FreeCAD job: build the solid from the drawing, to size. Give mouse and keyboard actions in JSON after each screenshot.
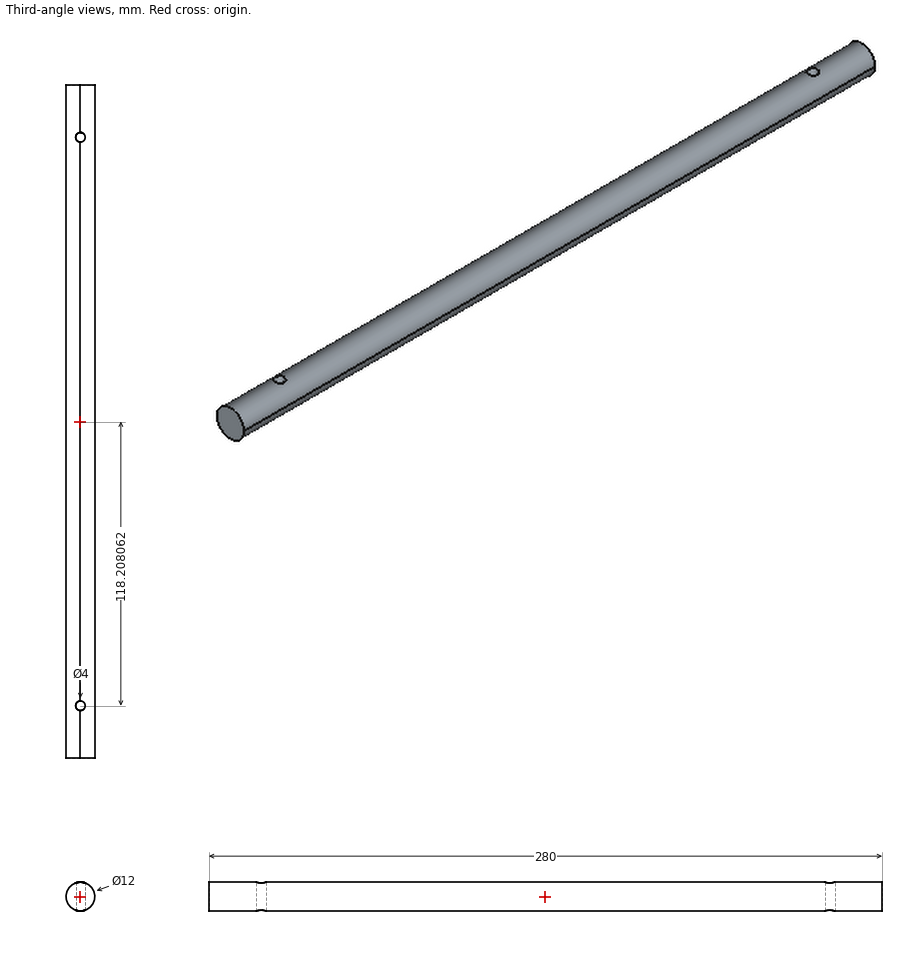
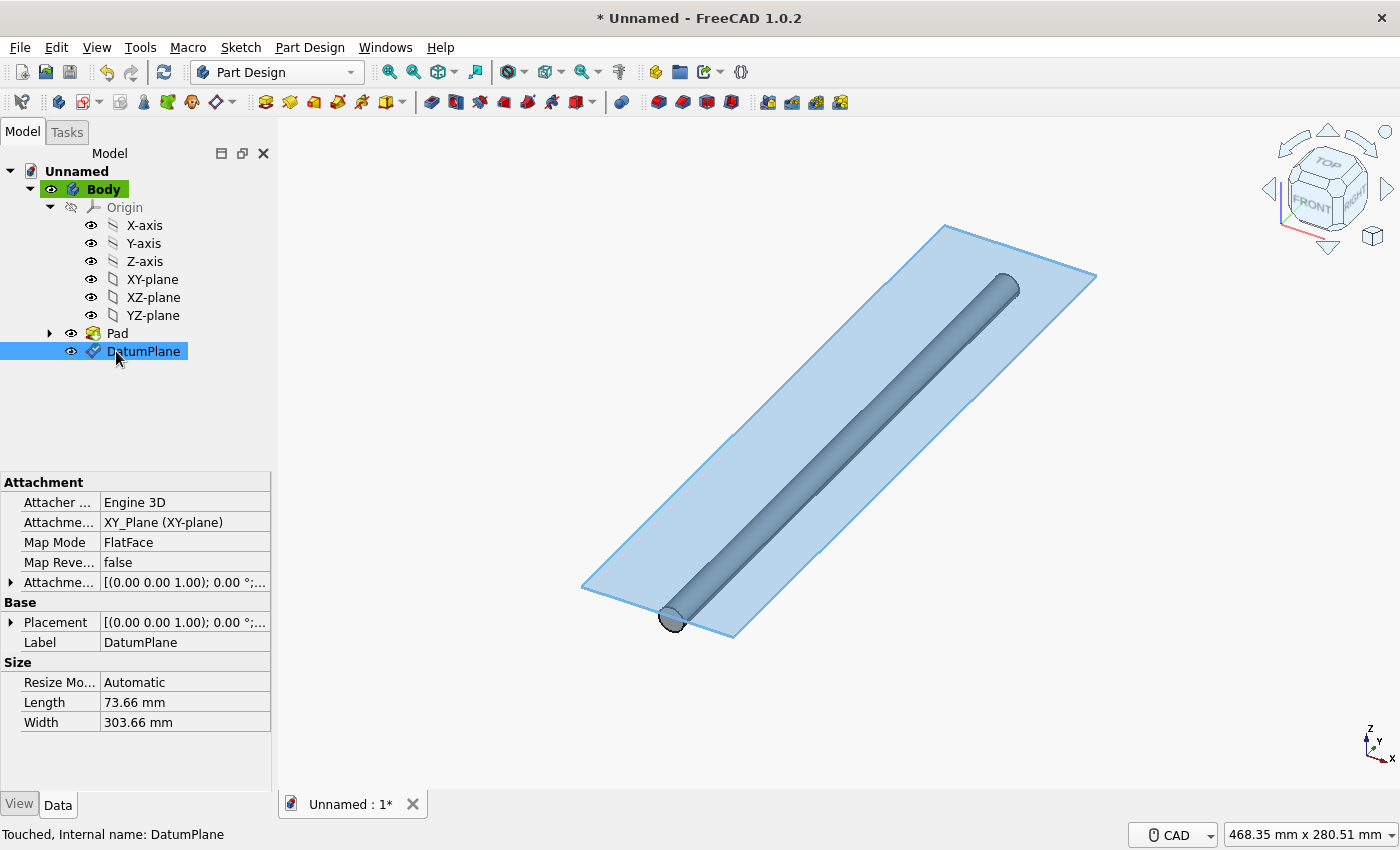
{"action": "left_click", "coordinate": [84, 102]}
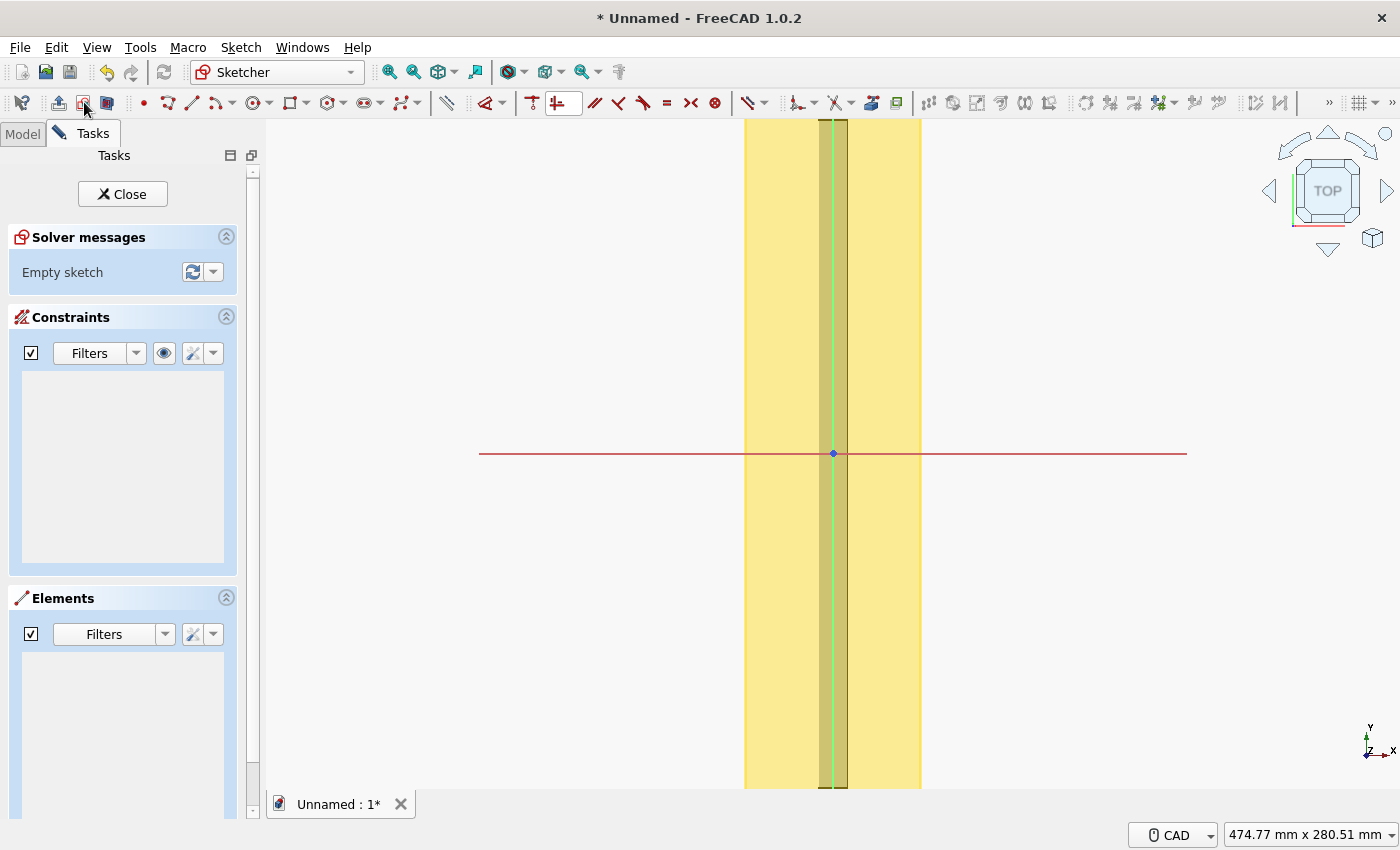
{"action": "scroll", "coordinate": [837, 751], "scroll_direction": "up", "scroll_amount": 15}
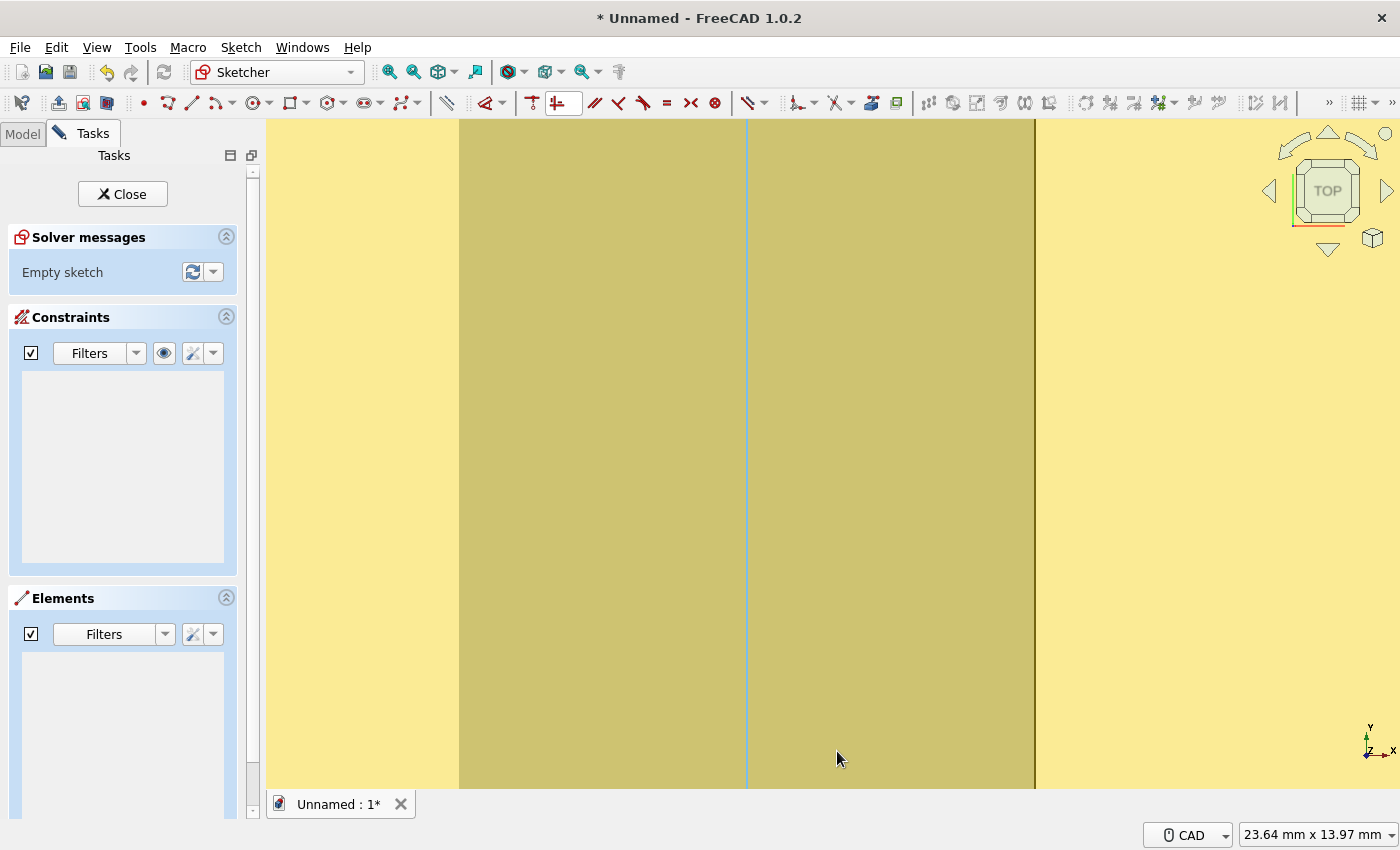
{"action": "scroll", "coordinate": [733, 426], "scroll_direction": "up", "scroll_amount": 4}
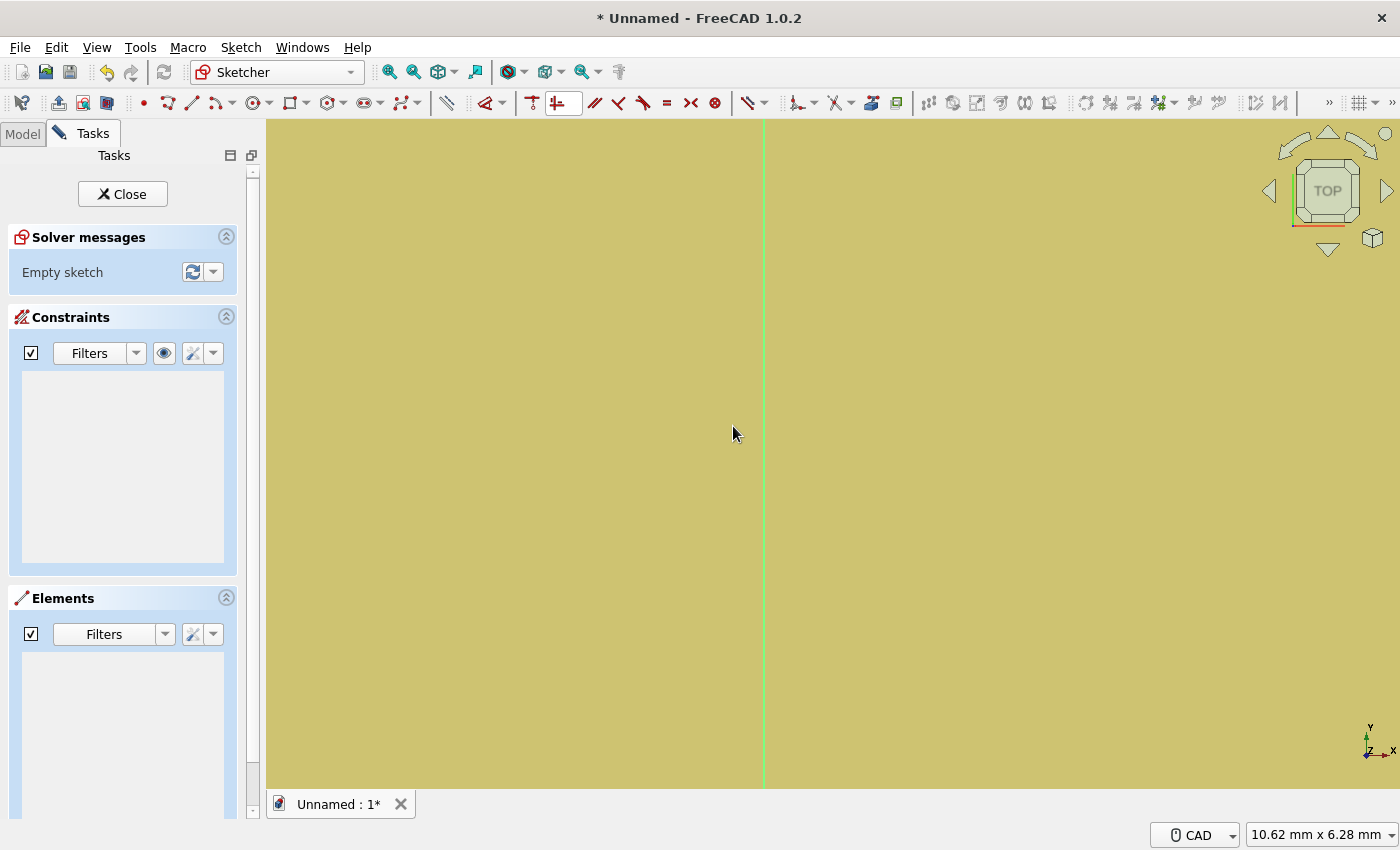
{"action": "left_click", "coordinate": [254, 104]}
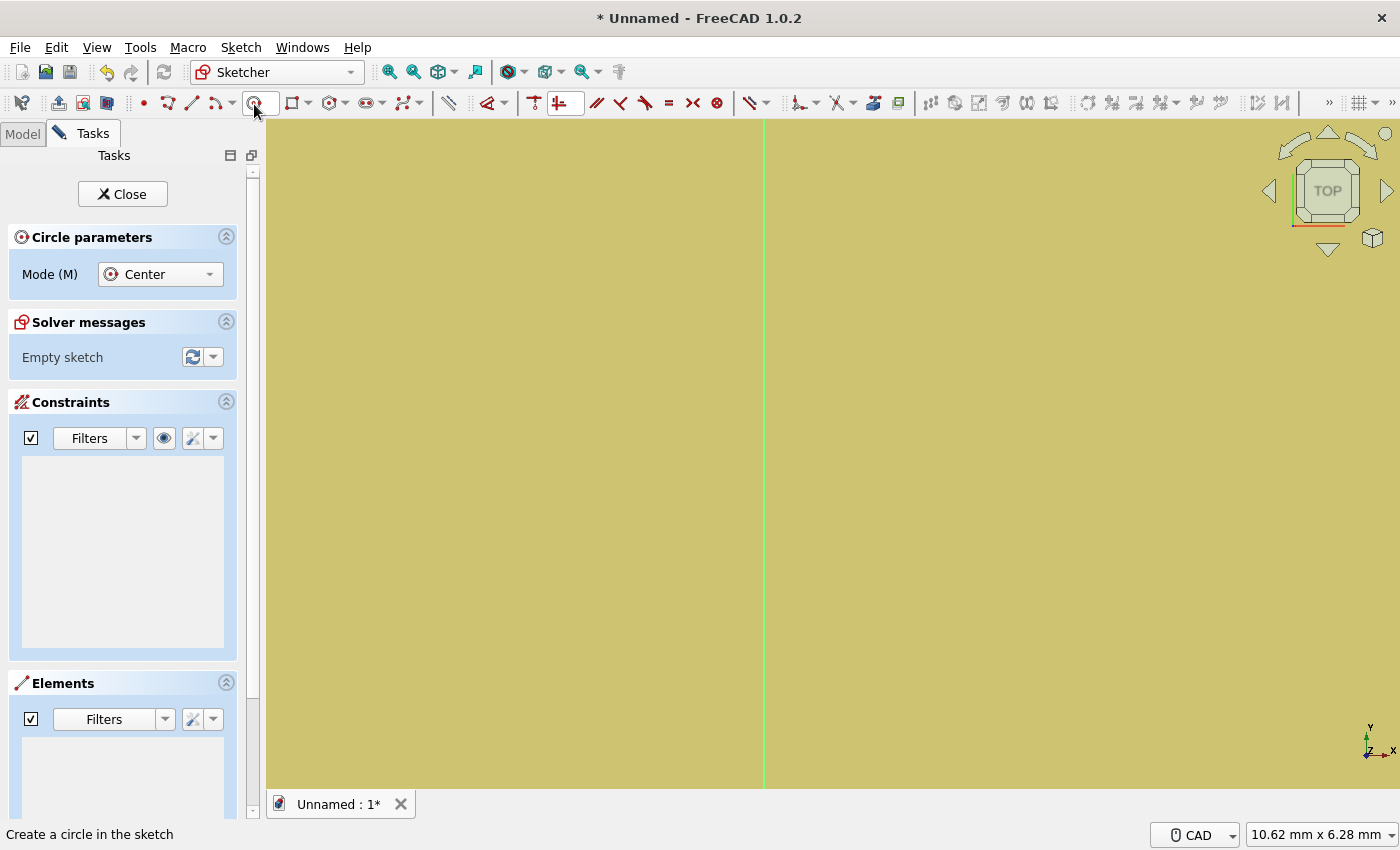
{"action": "left_click", "coordinate": [764, 453]}
{"action": "left_click", "coordinate": [915, 302]}
{"action": "key", "text": "Escape"}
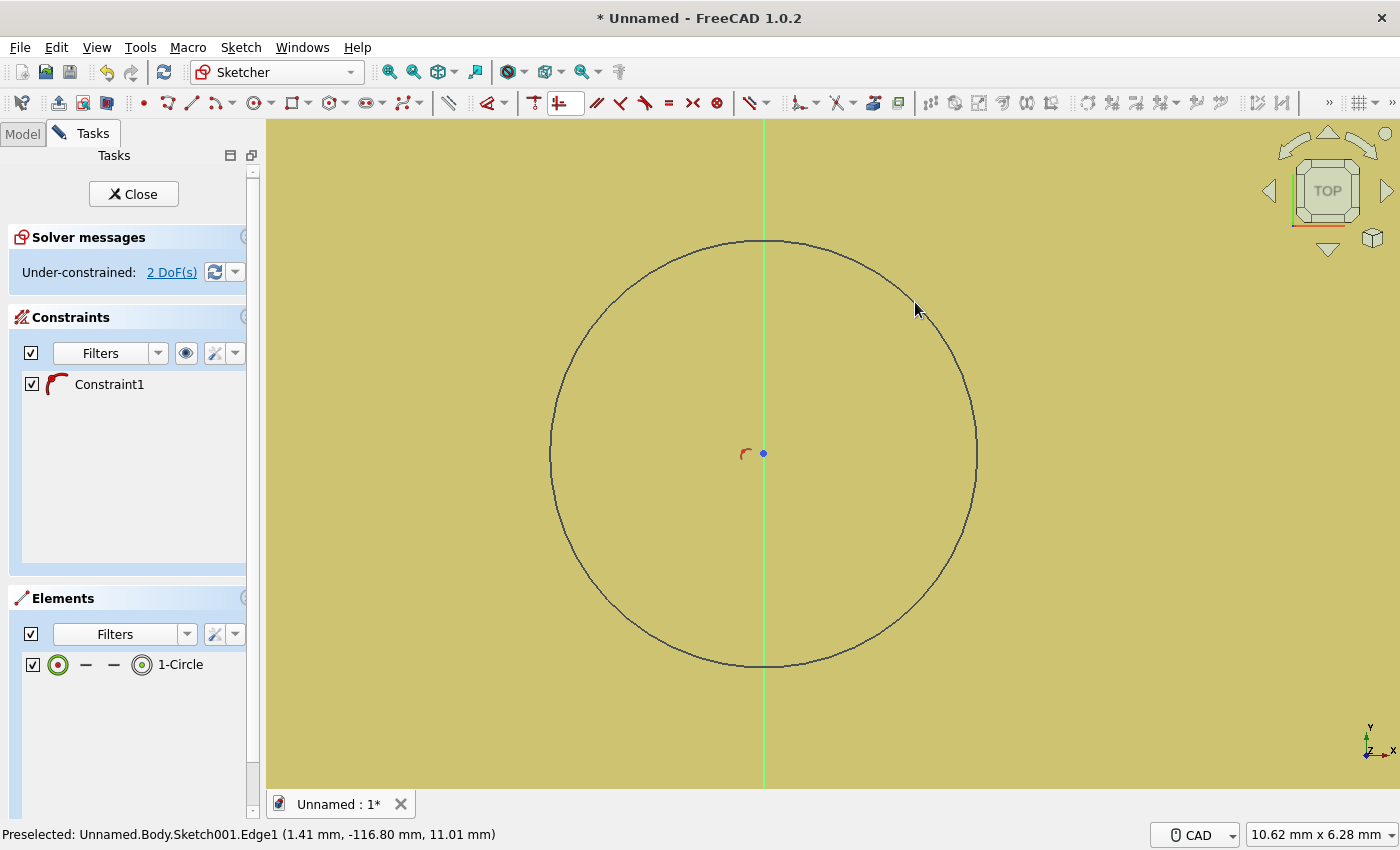
{"action": "left_click", "coordinate": [914, 302]}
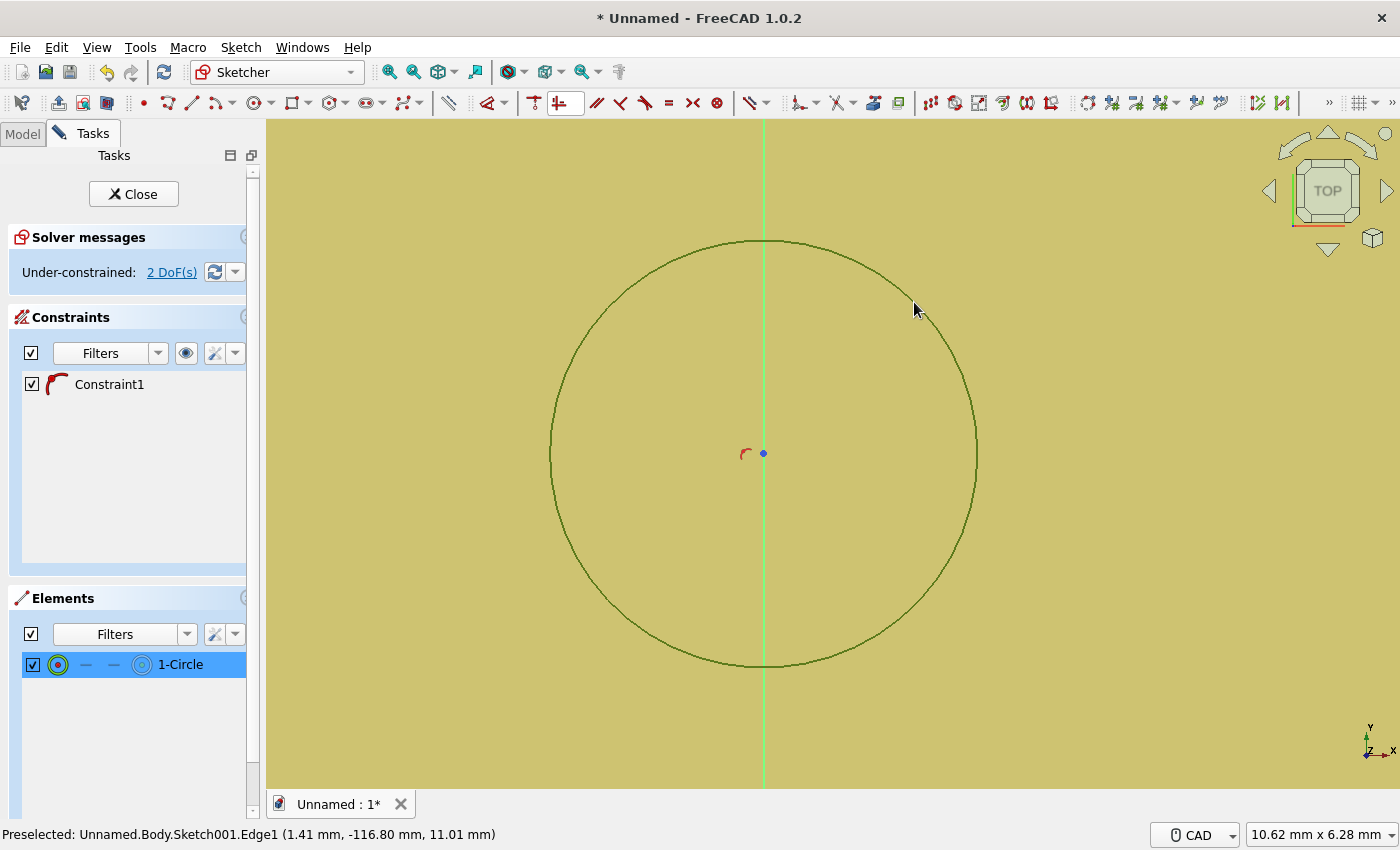
{"action": "key", "text": "k o"}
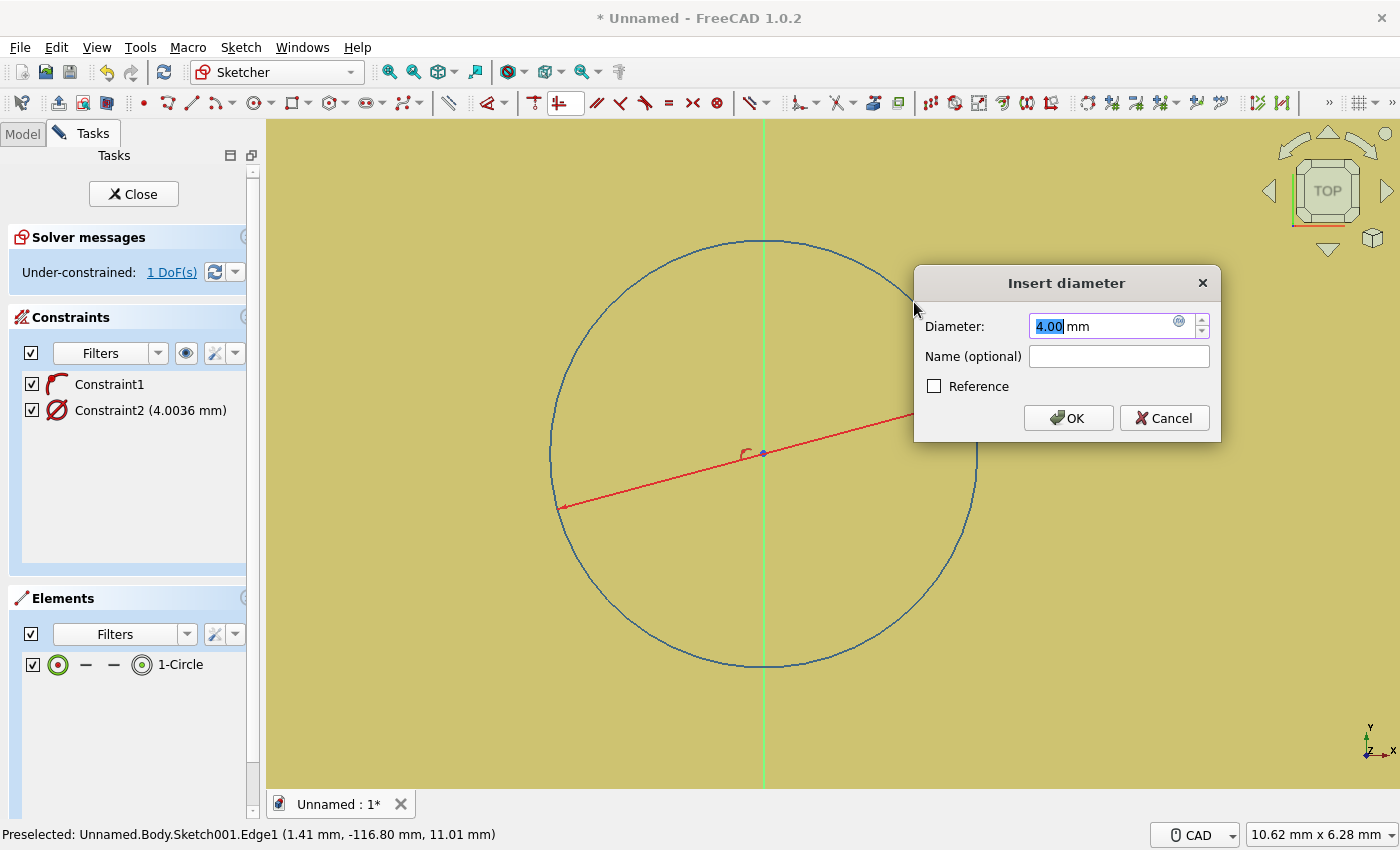
{"action": "type", "text": "4"}
{"action": "key", "text": "Return"}